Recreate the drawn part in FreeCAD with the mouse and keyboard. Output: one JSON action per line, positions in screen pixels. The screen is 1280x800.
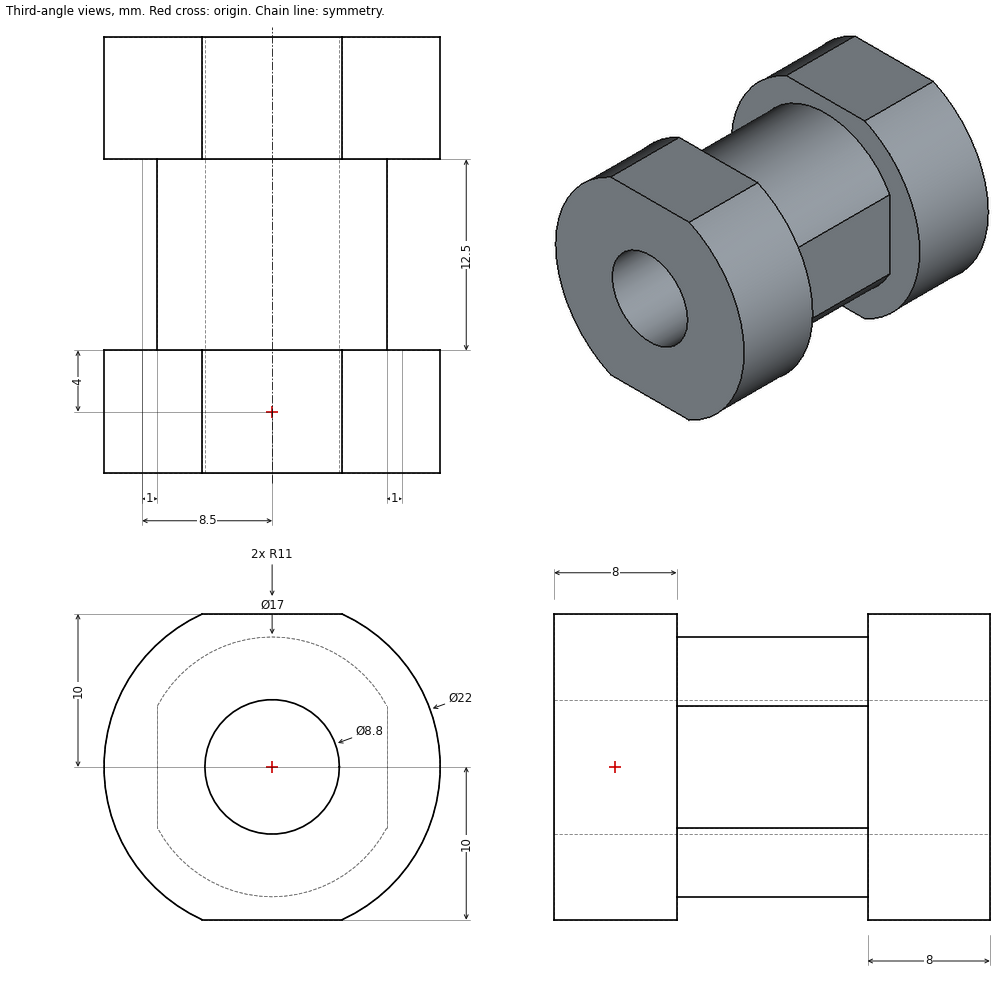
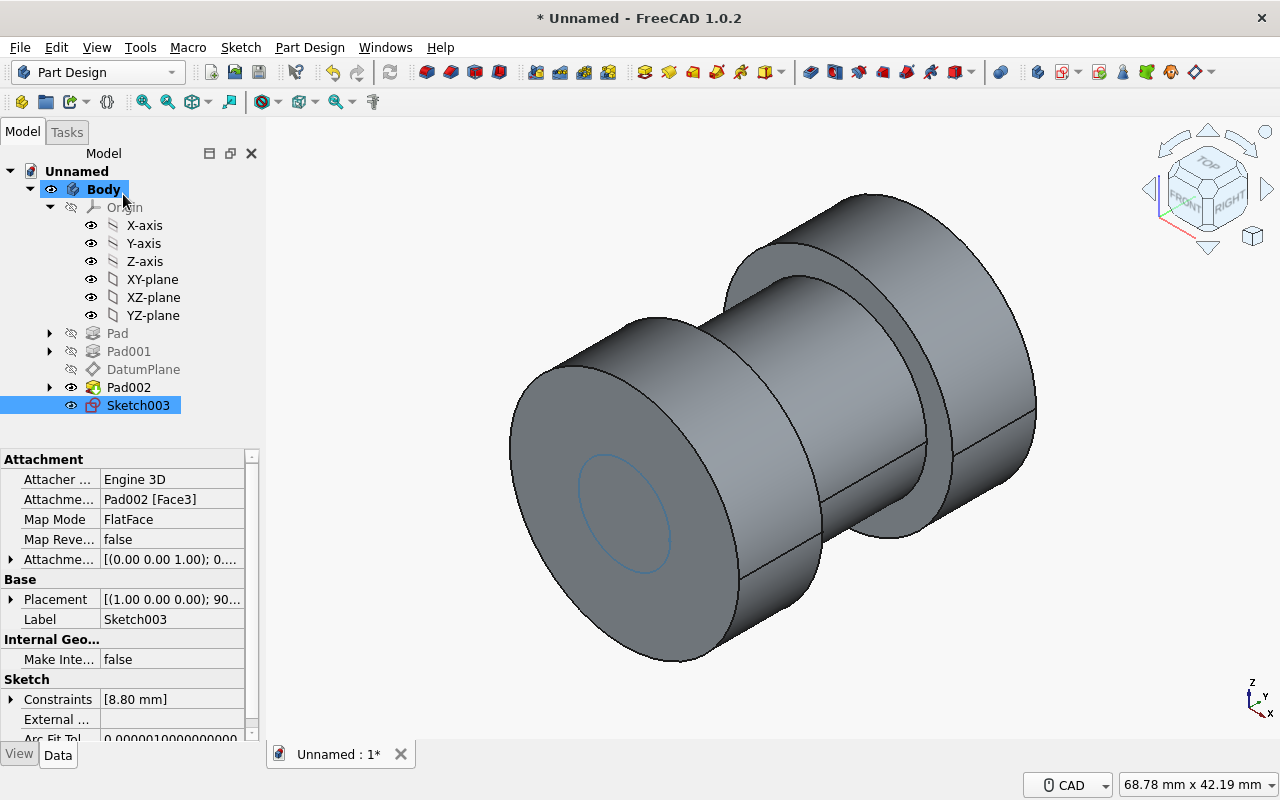
{"action": "left_click", "coordinate": [812, 72]}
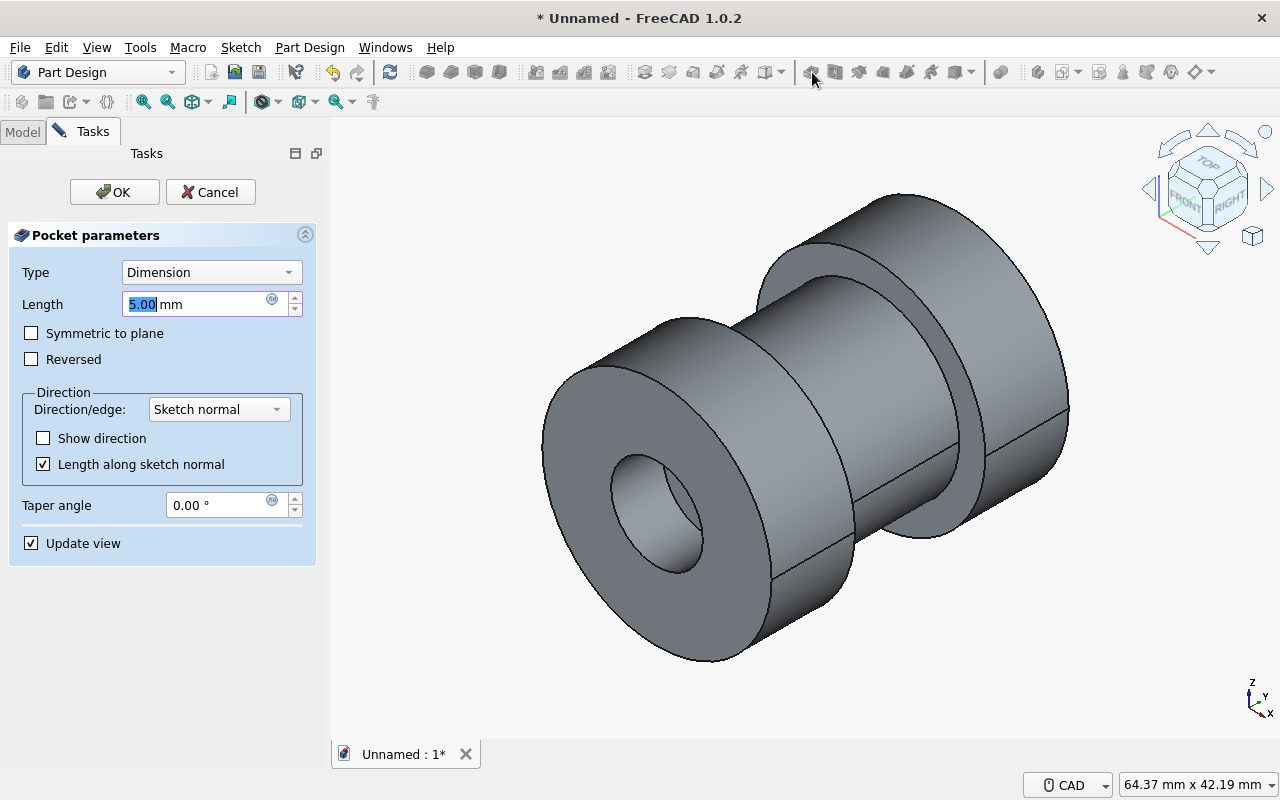
{"action": "left_click", "coordinate": [212, 272]}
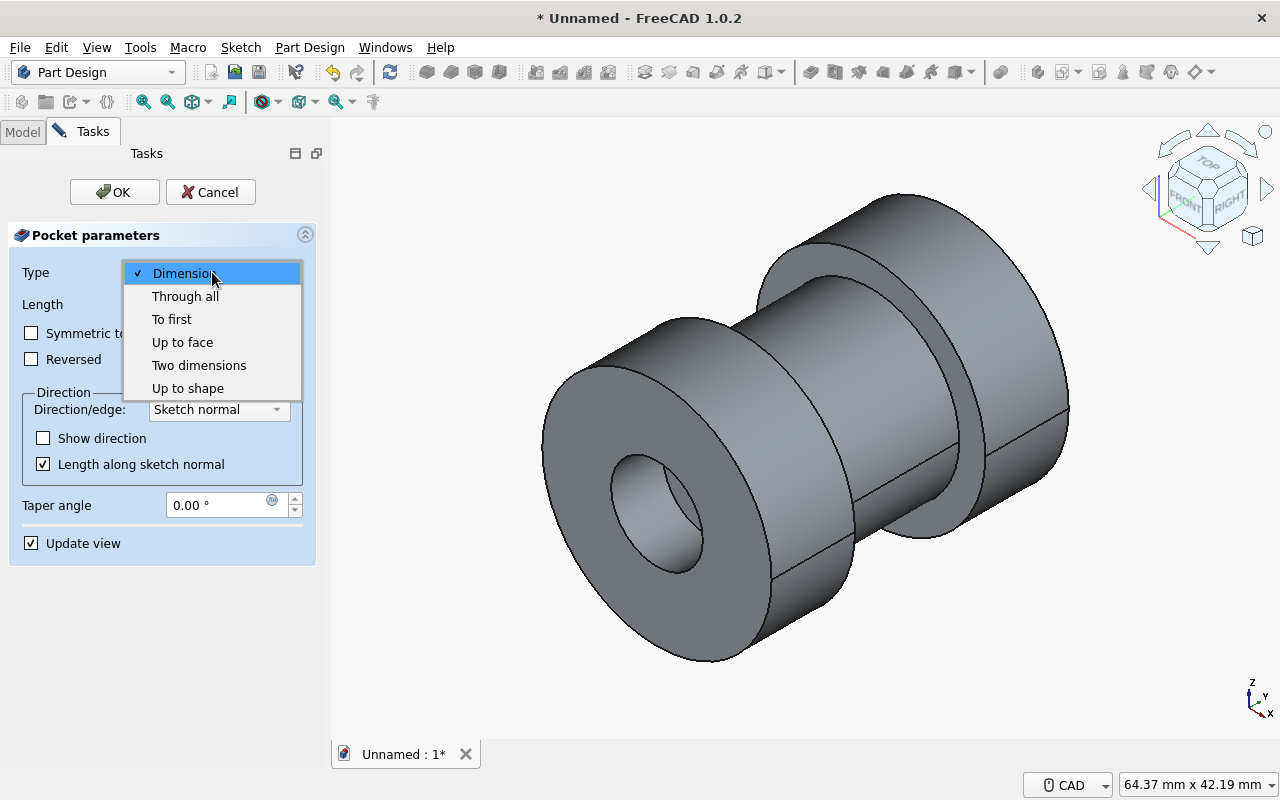
{"action": "left_click", "coordinate": [212, 296]}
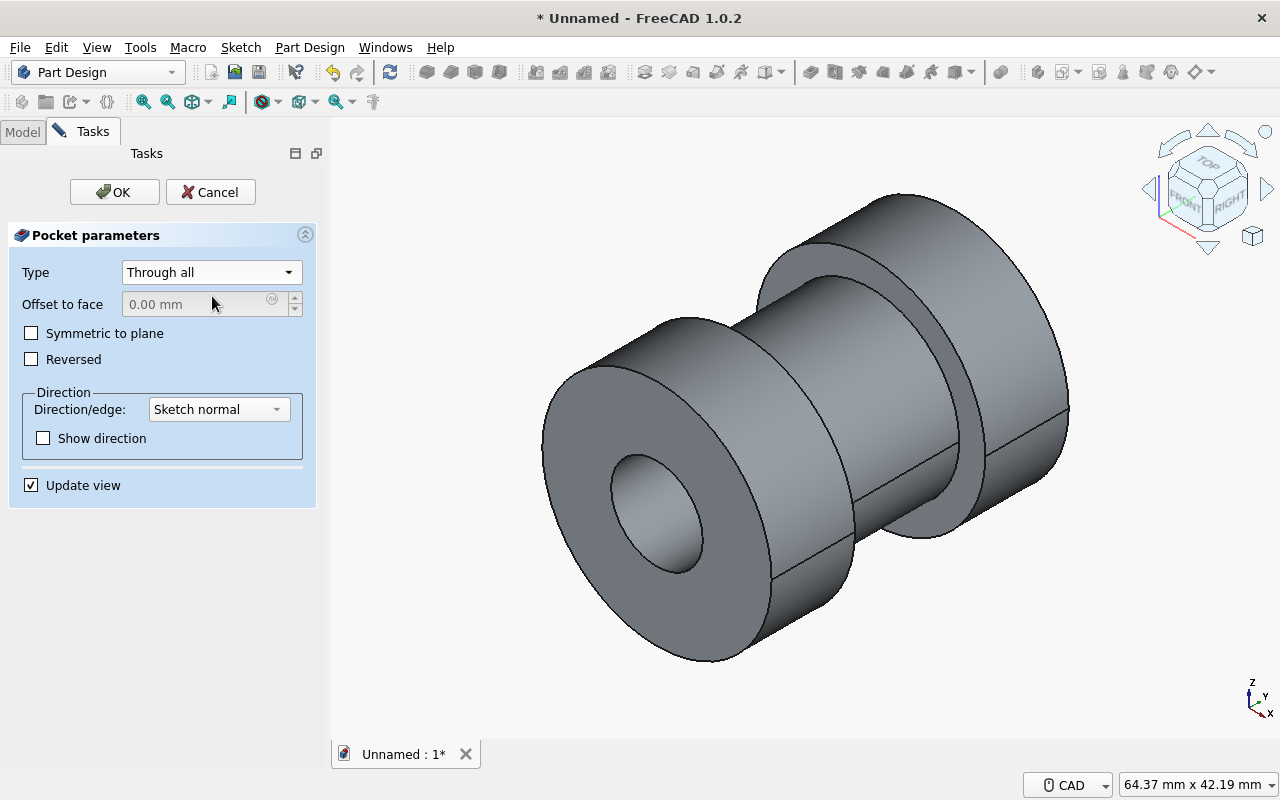
{"action": "left_click", "coordinate": [115, 192]}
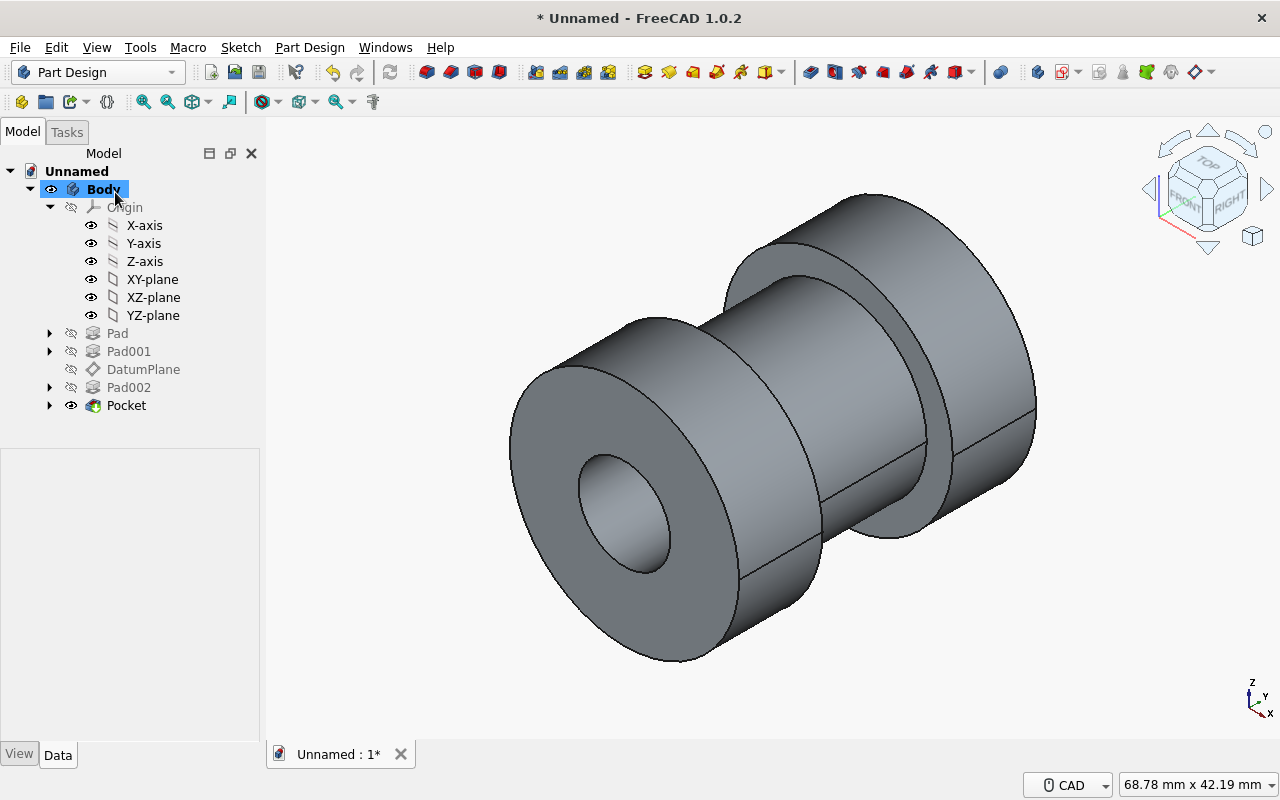
{"action": "left_click", "coordinate": [592, 570]}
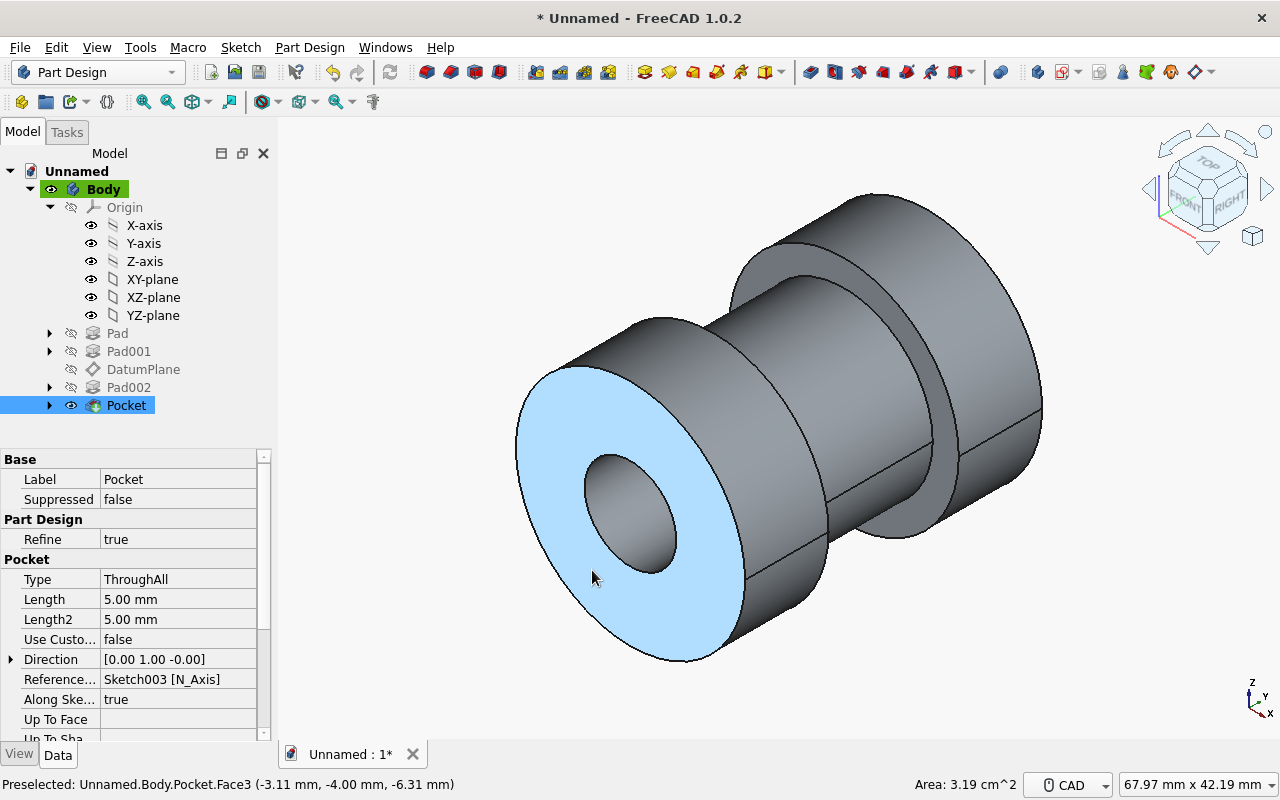
{"action": "left_click", "coordinate": [1062, 72]}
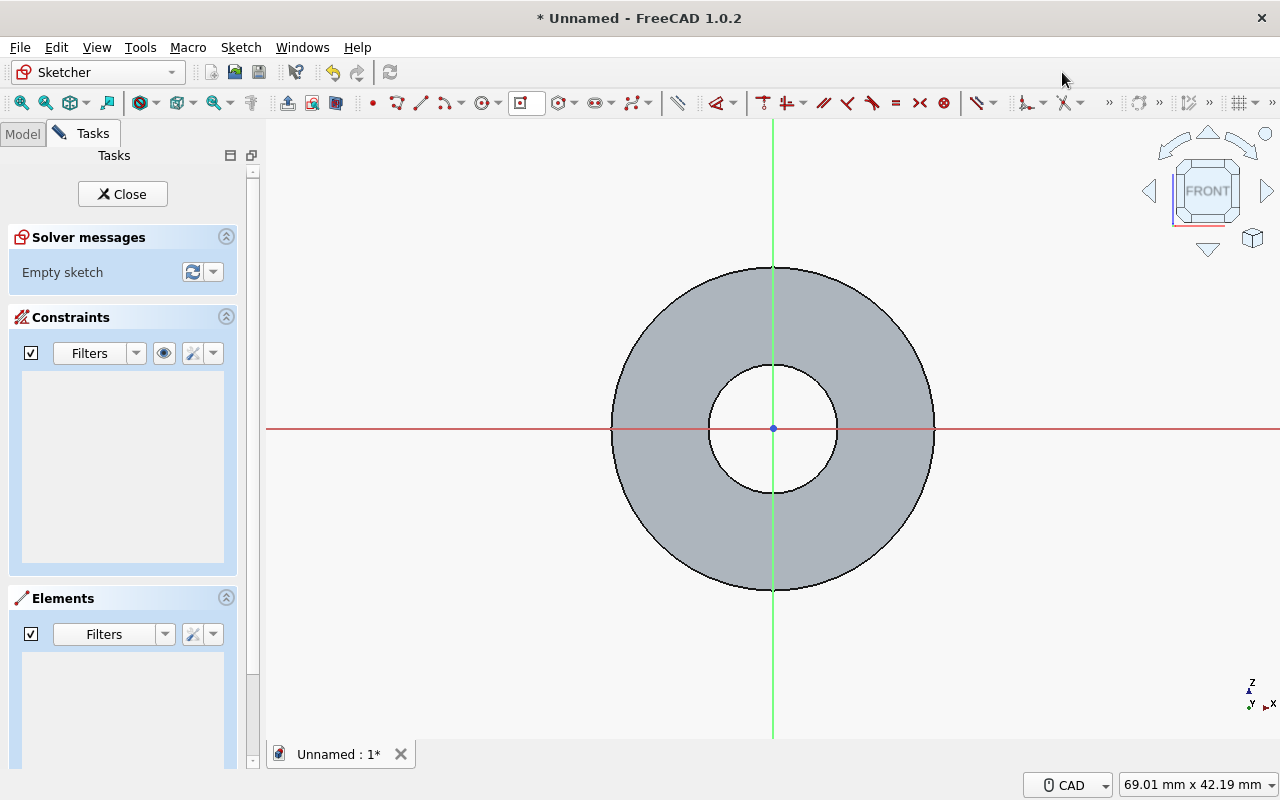
{"action": "key", "text": "g l"}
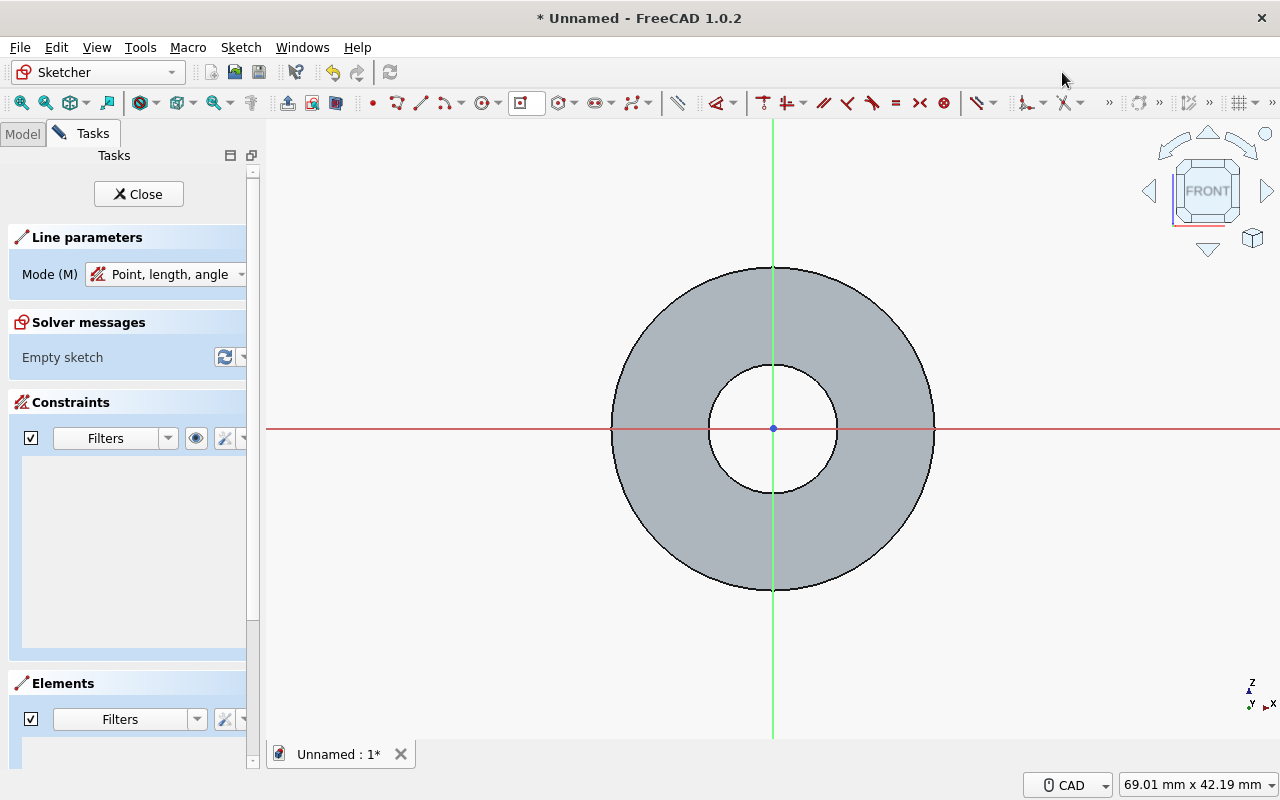
{"action": "left_click", "coordinate": [706, 282]}
{"action": "left_click", "coordinate": [840, 282]}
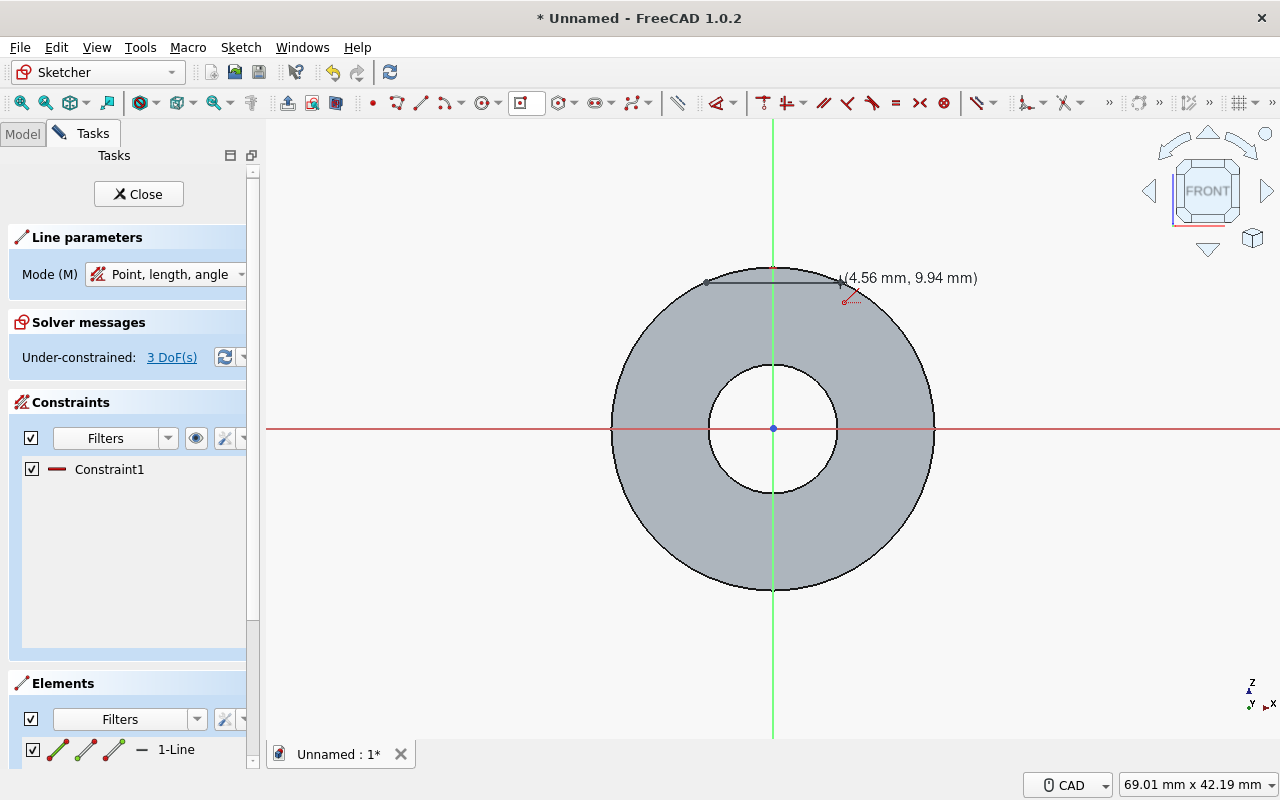
{"action": "key", "text": "g 3 a"}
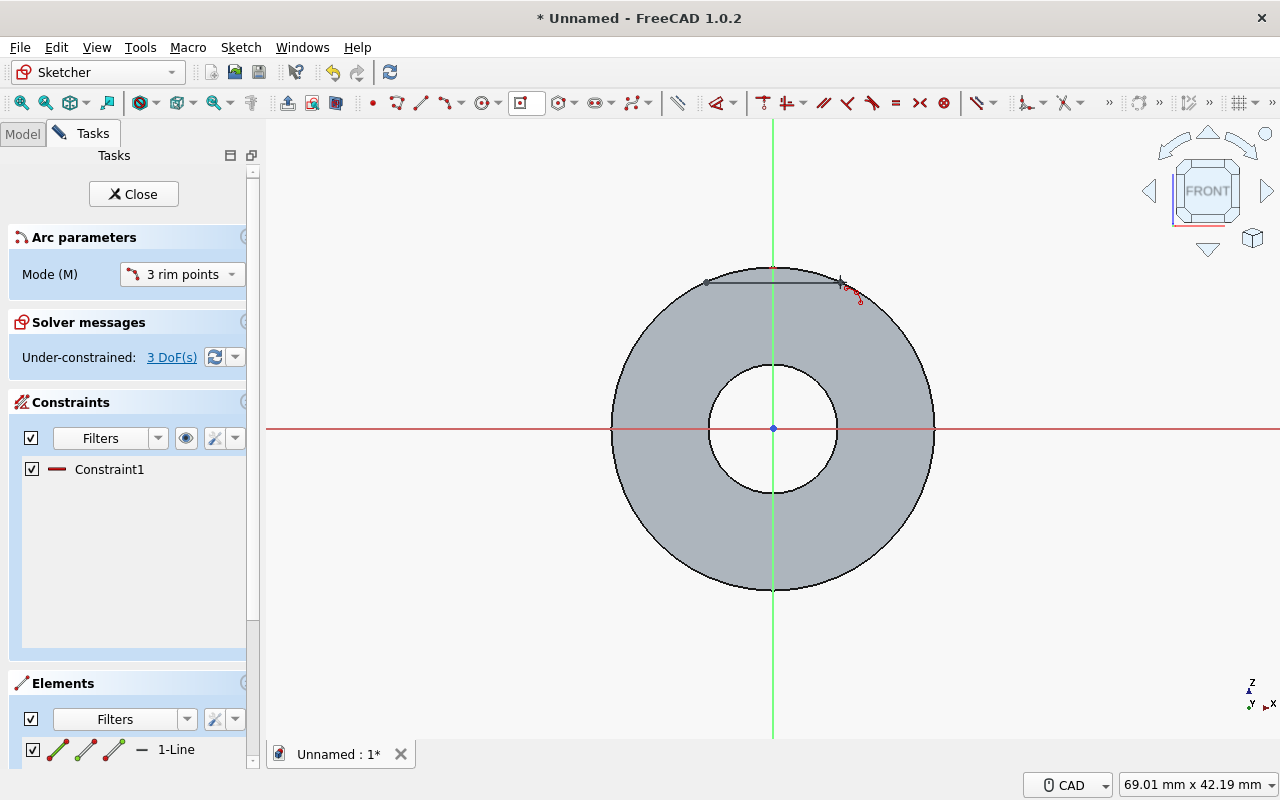
{"action": "left_click", "coordinate": [840, 283]}
{"action": "left_click", "coordinate": [706, 283]}
{"action": "left_click", "coordinate": [787, 268]}